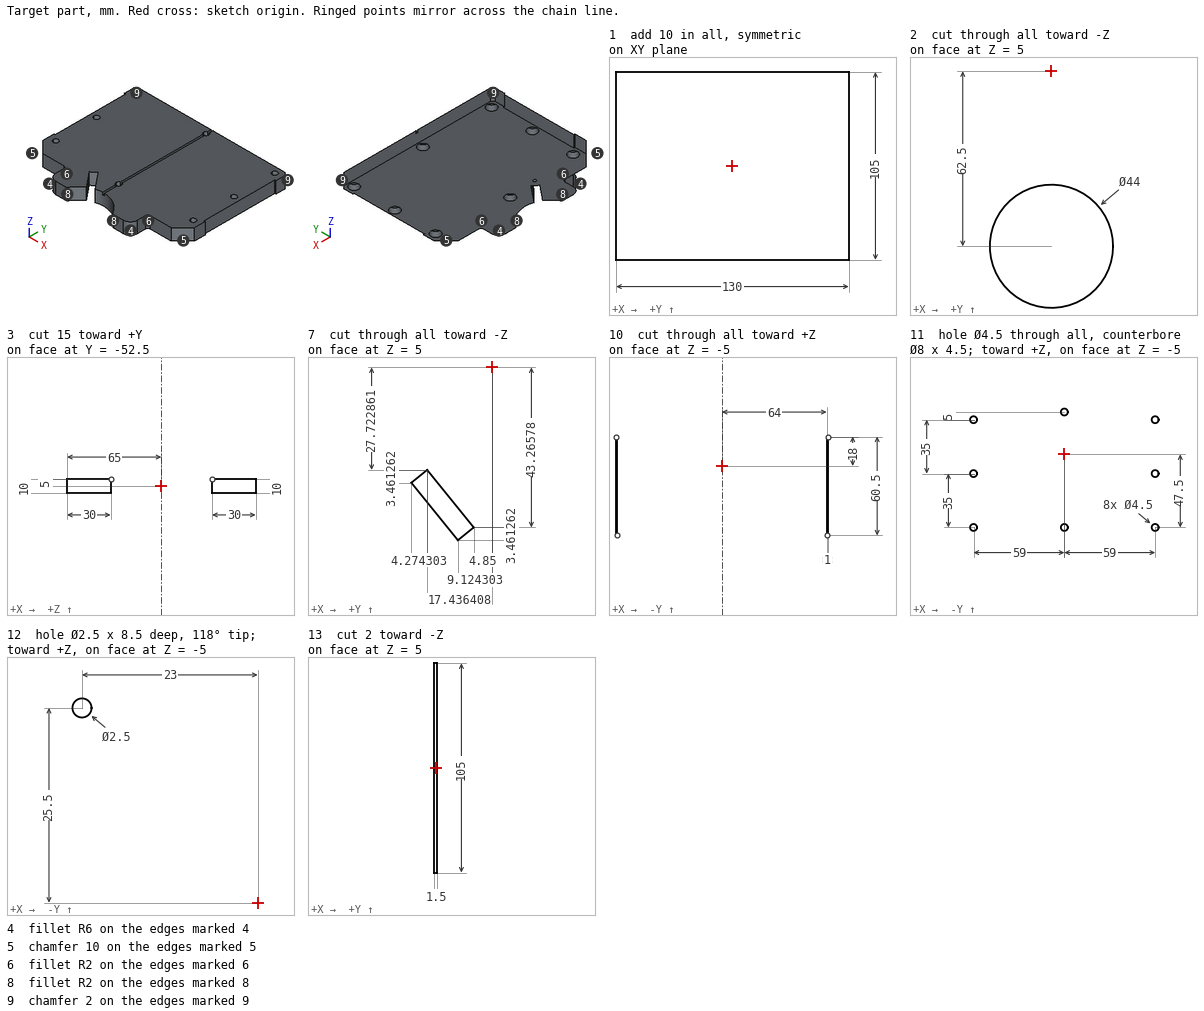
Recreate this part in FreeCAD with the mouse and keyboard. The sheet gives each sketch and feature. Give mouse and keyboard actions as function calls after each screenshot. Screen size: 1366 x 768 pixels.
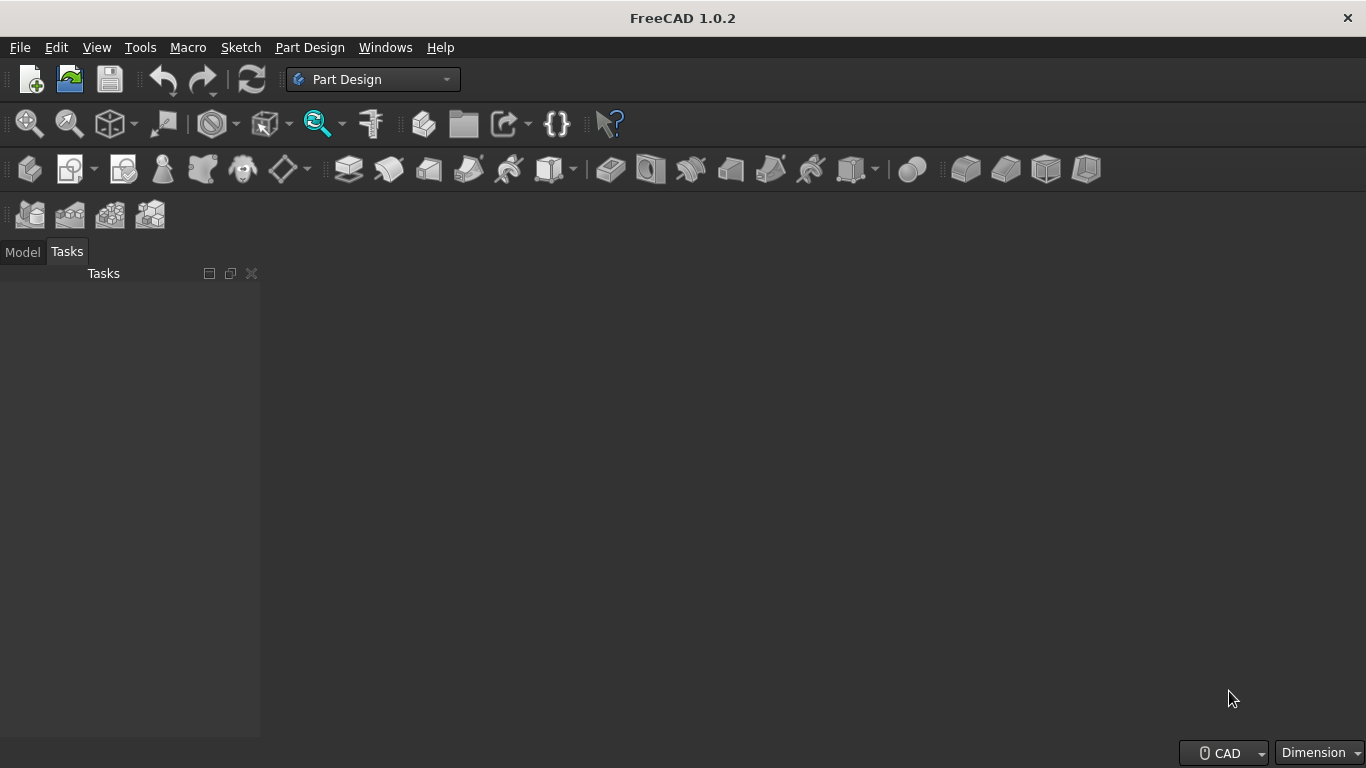
click(30, 80)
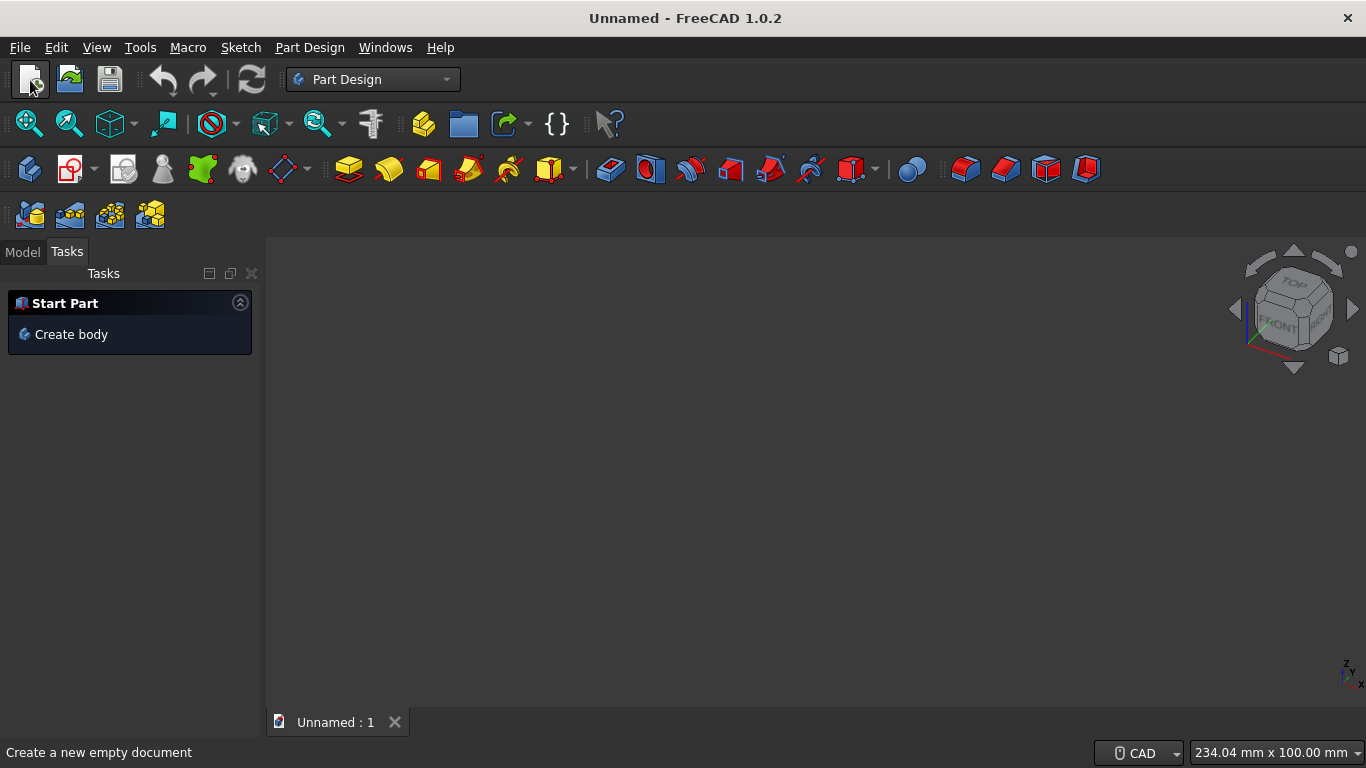
click(70, 170)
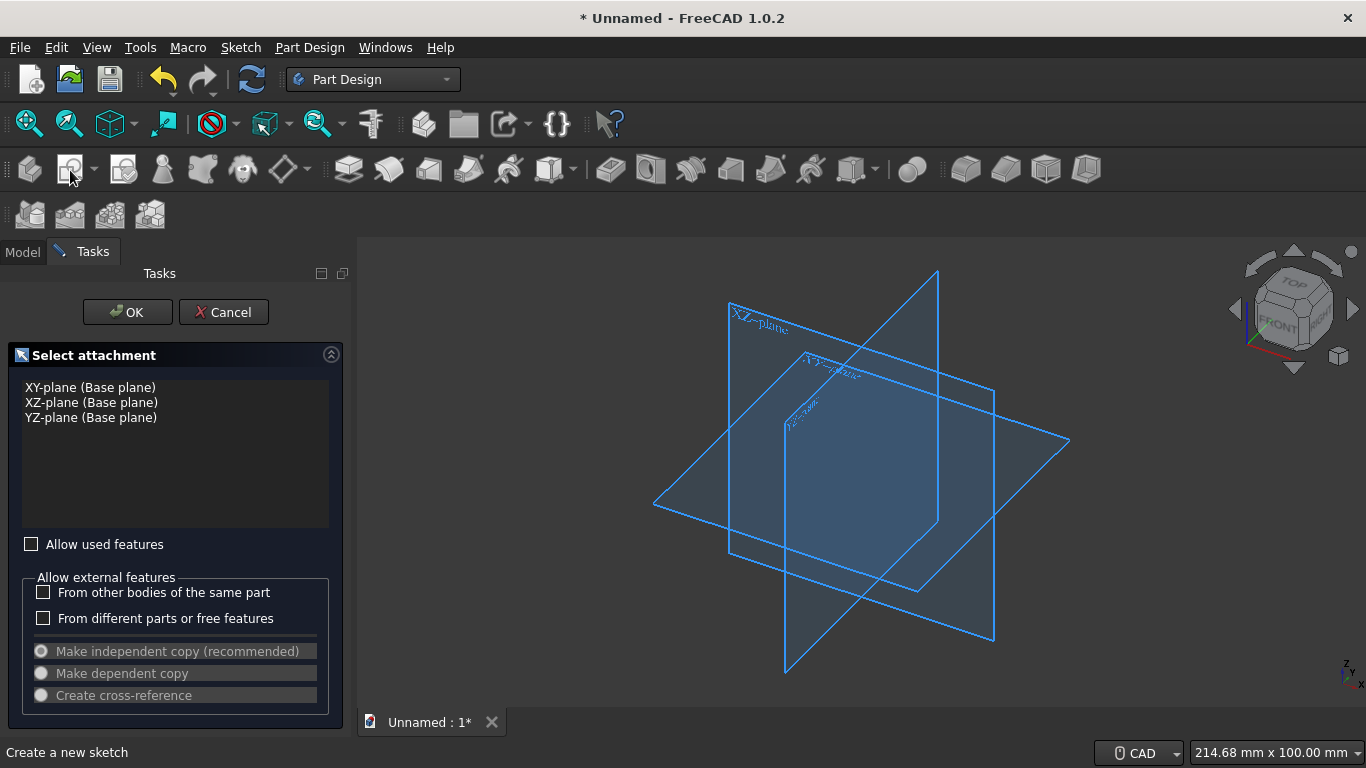
click(82, 388)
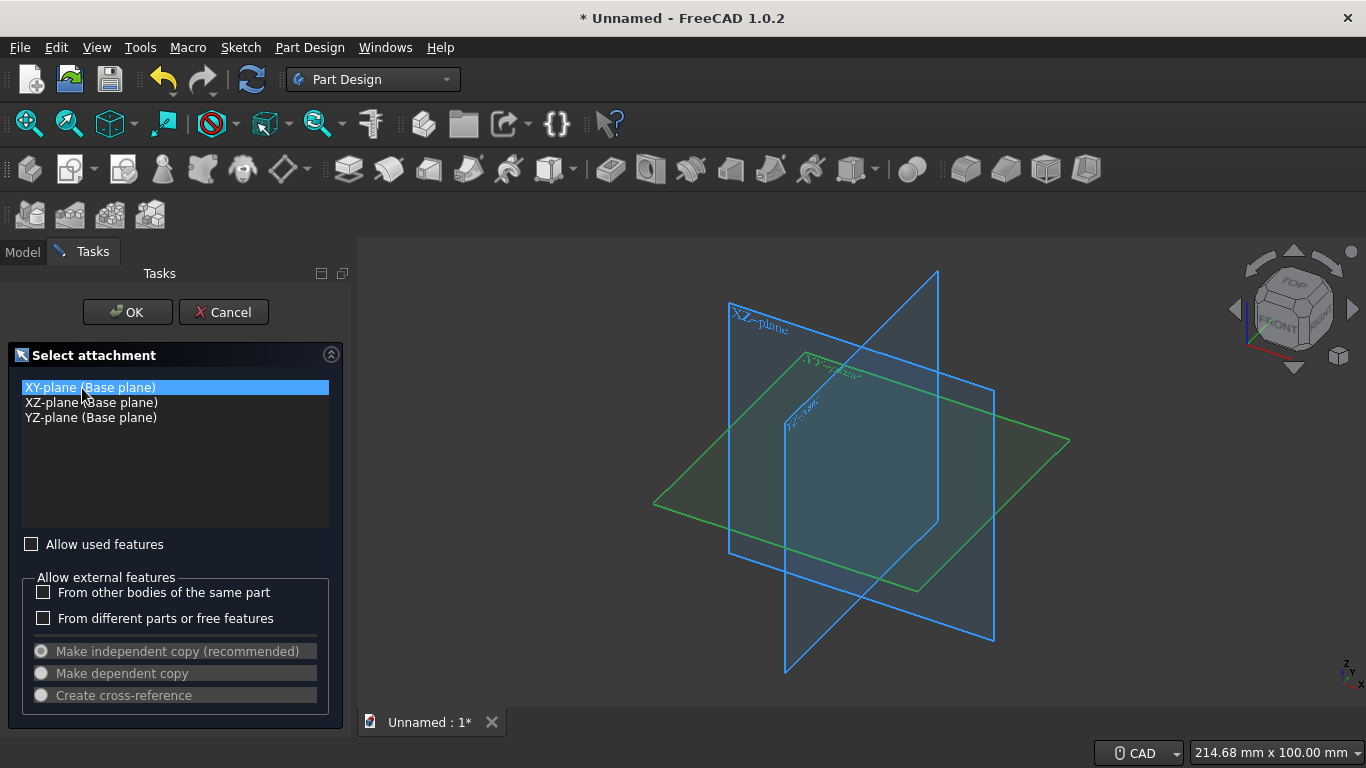
click(128, 312)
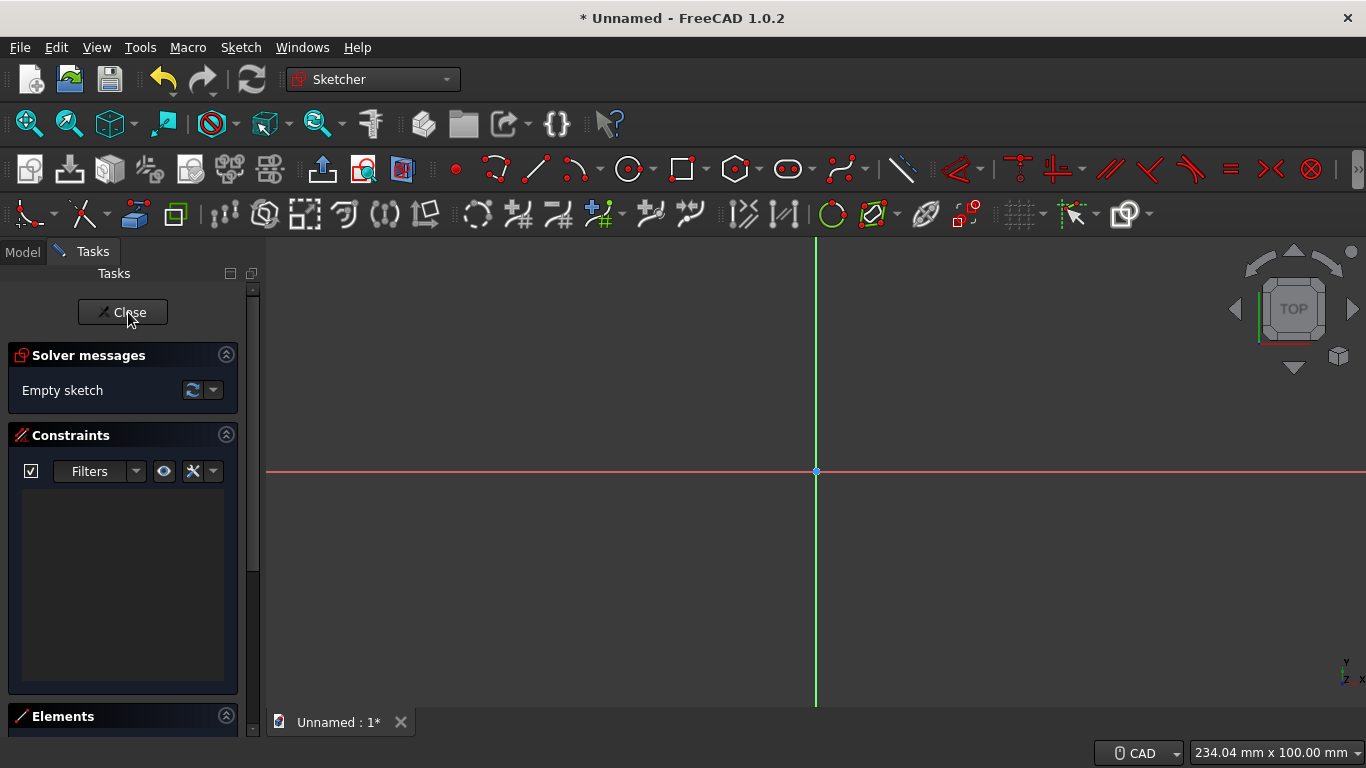
scroll(664, 472, down, 3)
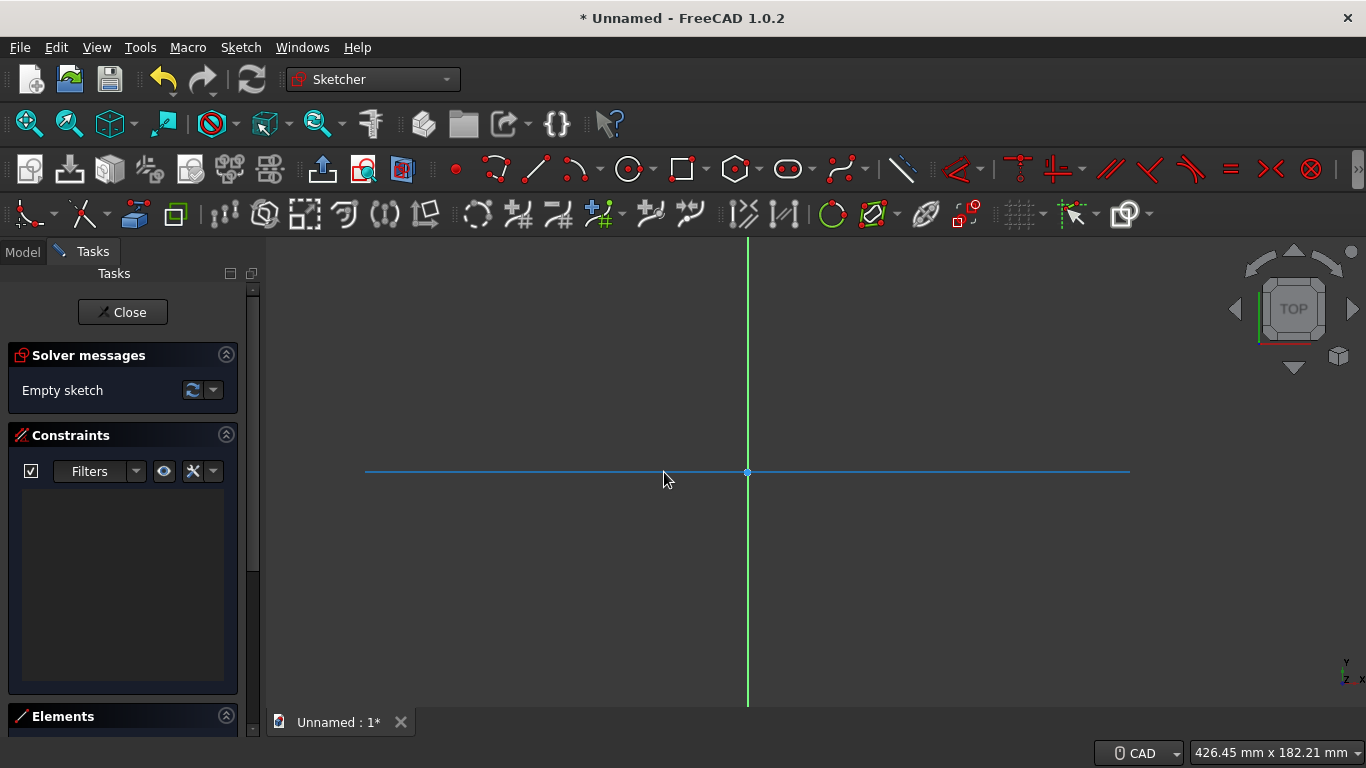
key(g)
key(v)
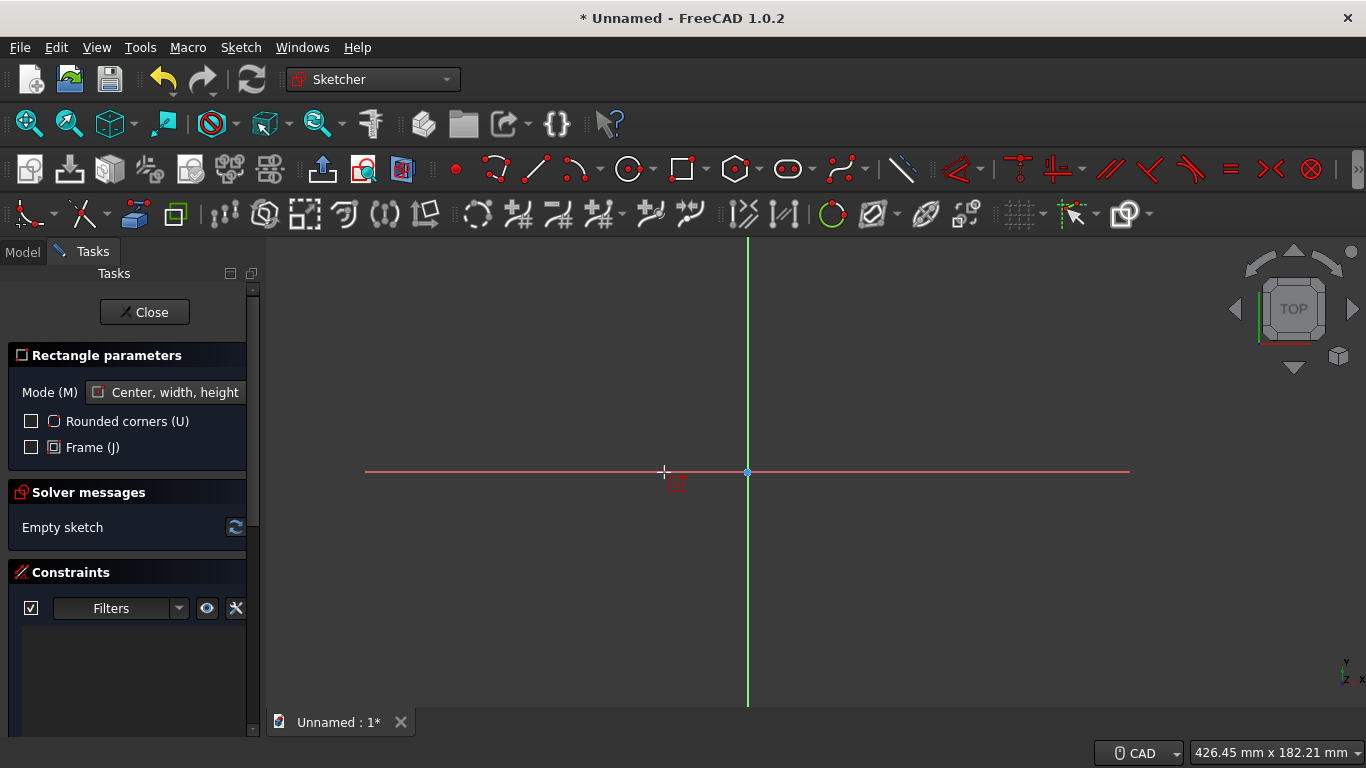
click(748, 472)
move(915, 337)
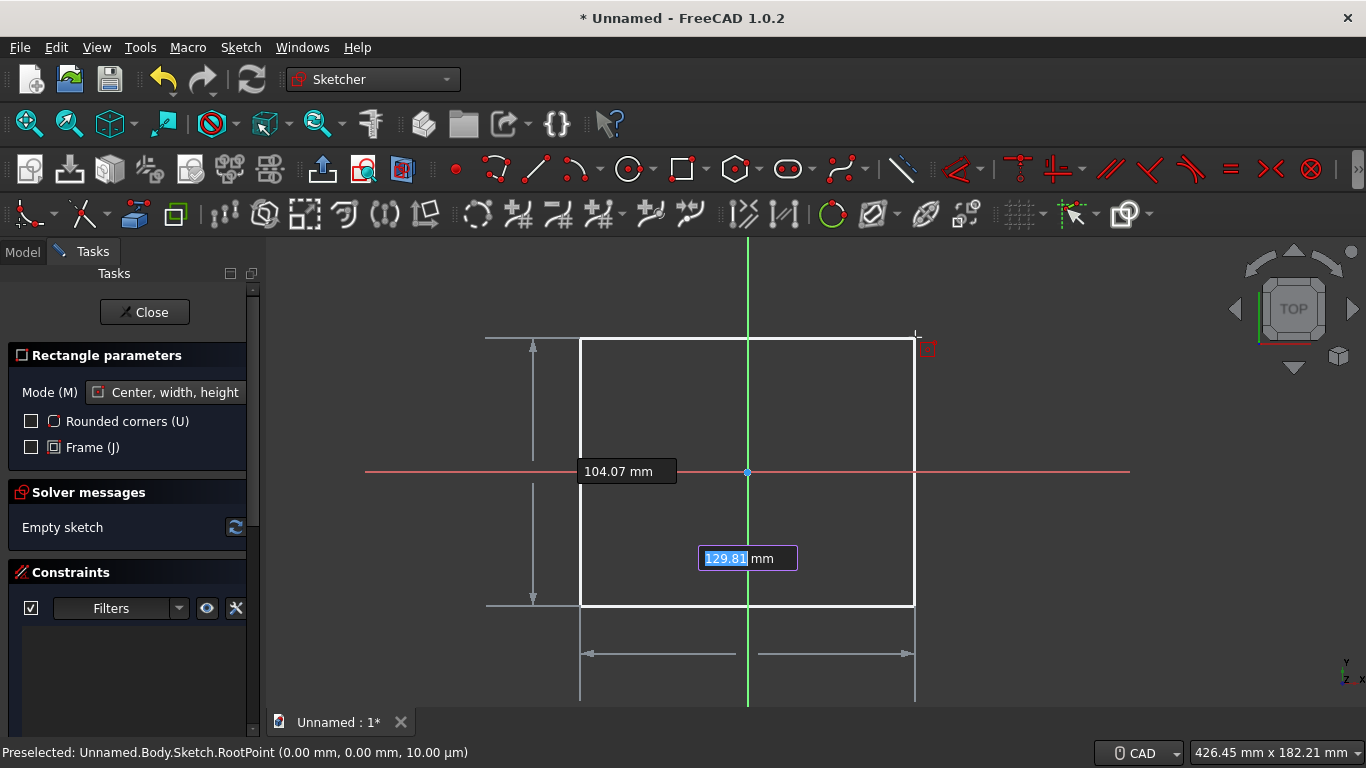
text(130)
key(Tab)
text(105)
key(Return)
key(Escape)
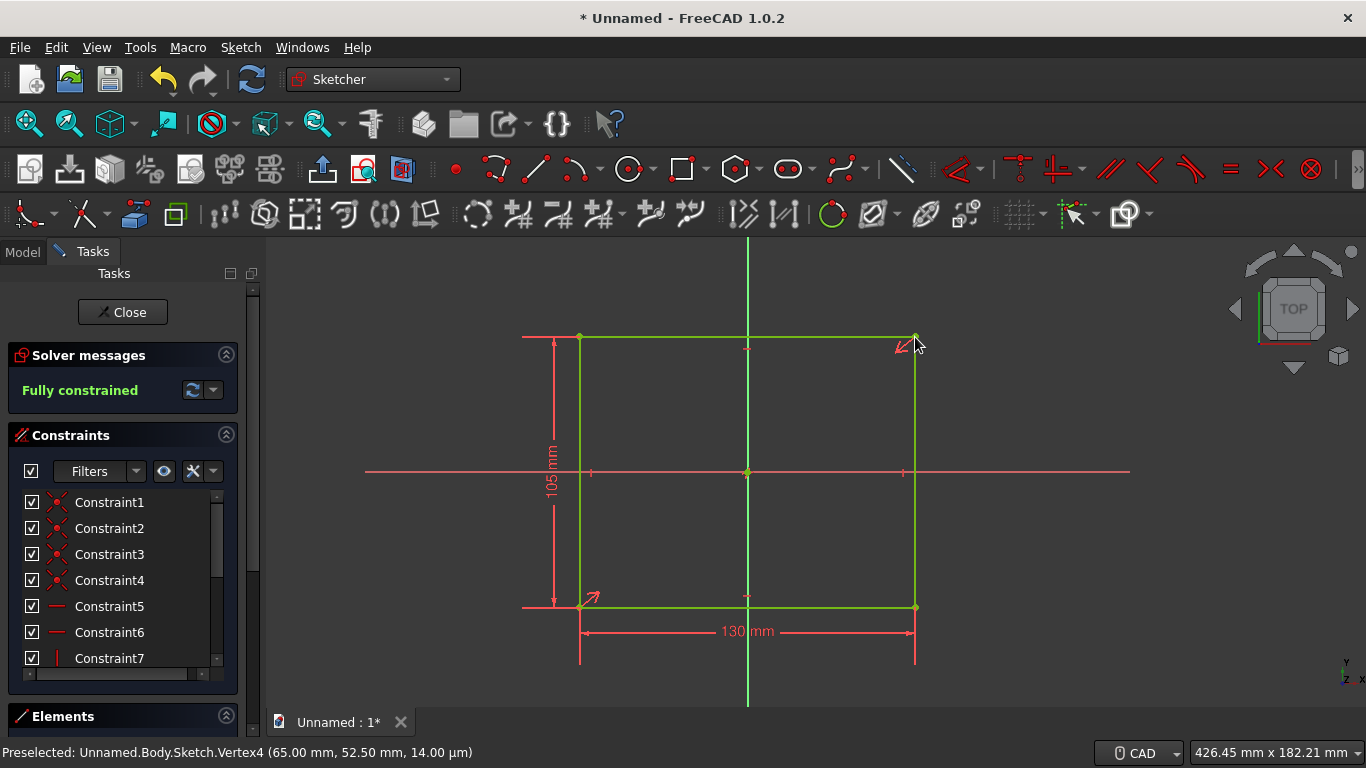
click(123, 312)